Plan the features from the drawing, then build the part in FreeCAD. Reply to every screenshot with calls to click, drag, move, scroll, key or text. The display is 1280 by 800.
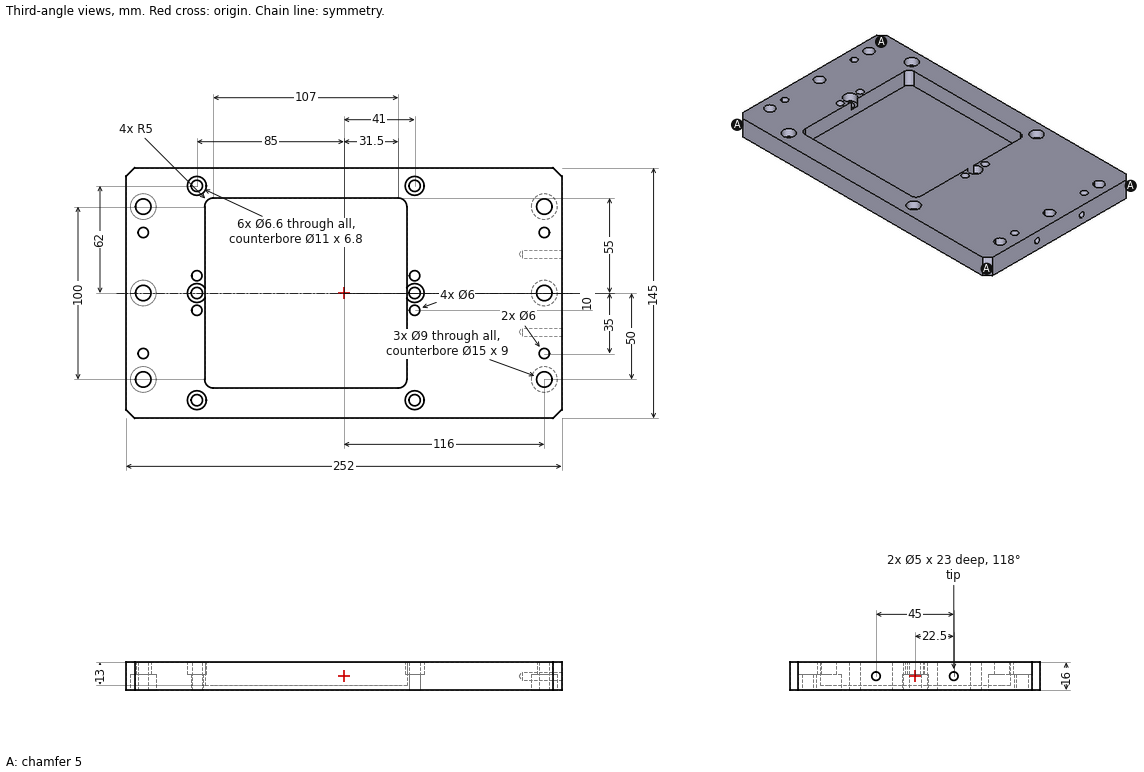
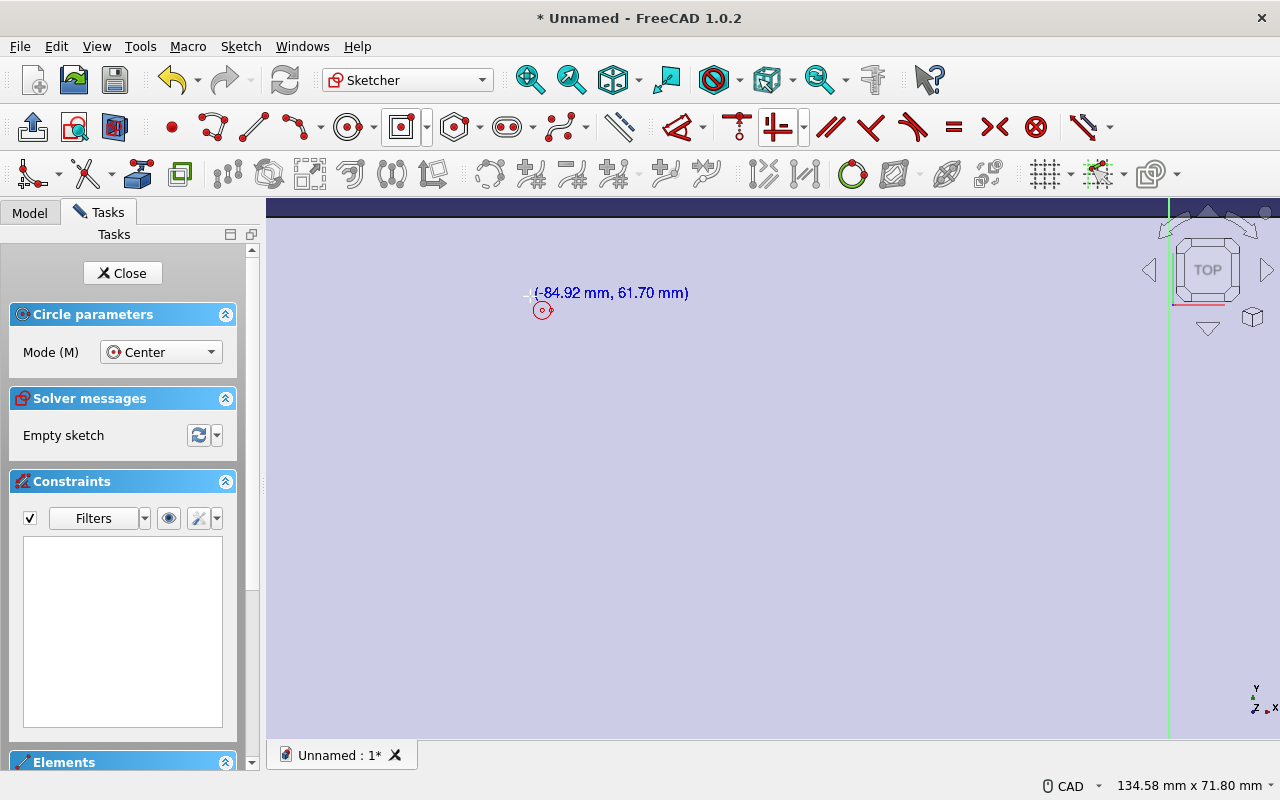
click(529, 296)
move(547, 279)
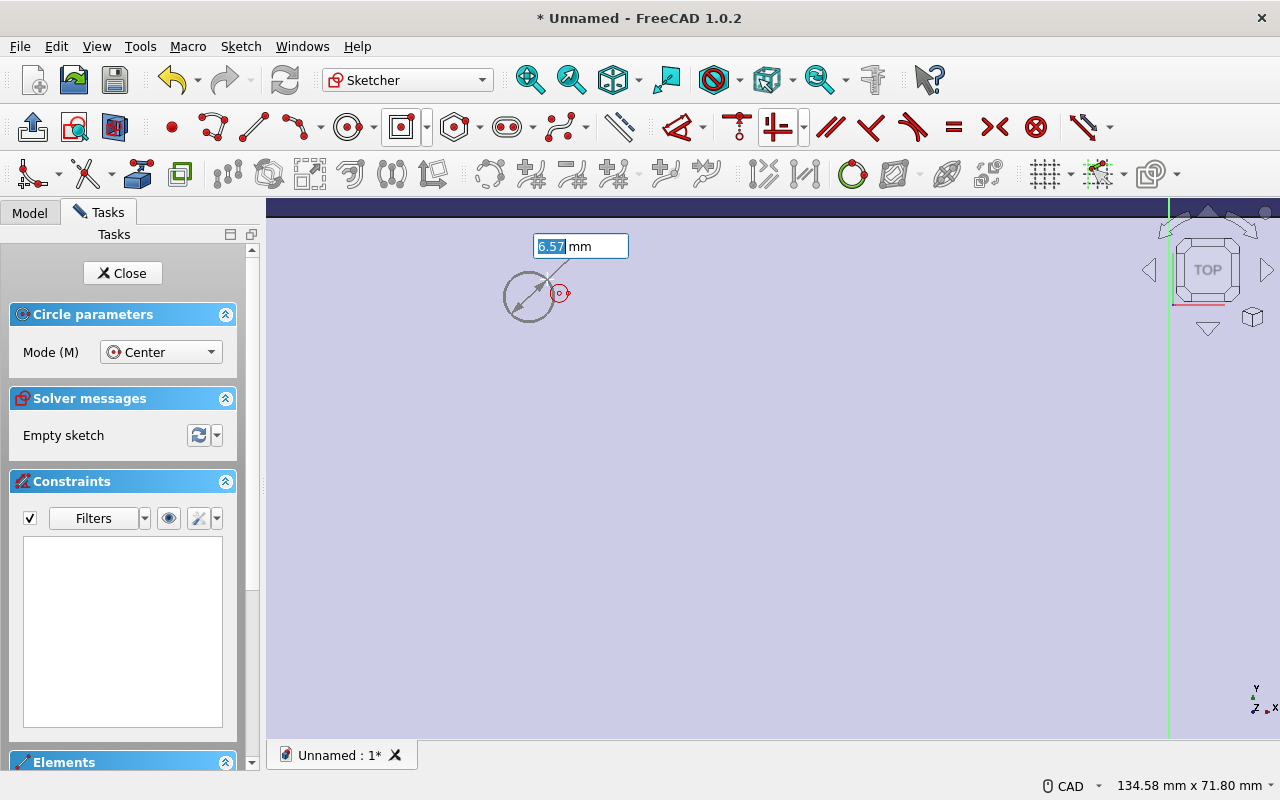
text(6.6)
key(Return)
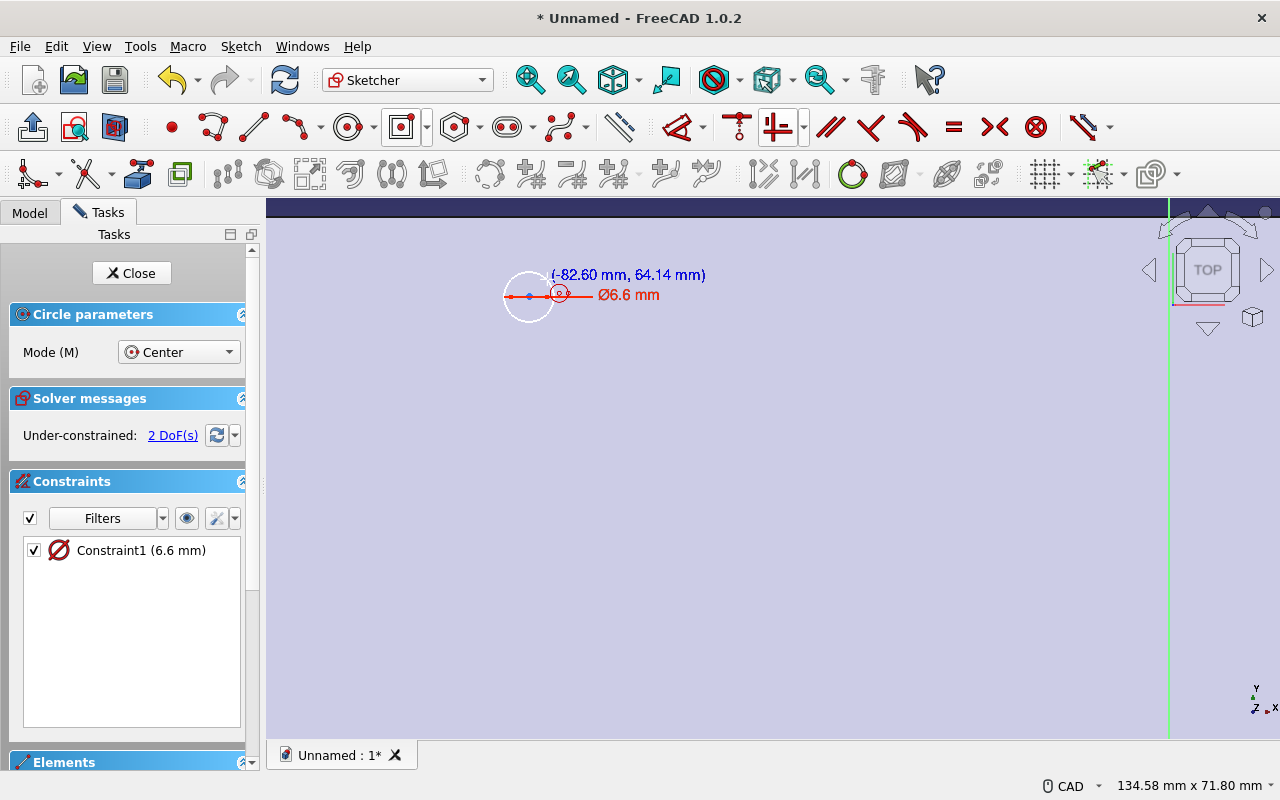
scroll(530, 297, down, 5)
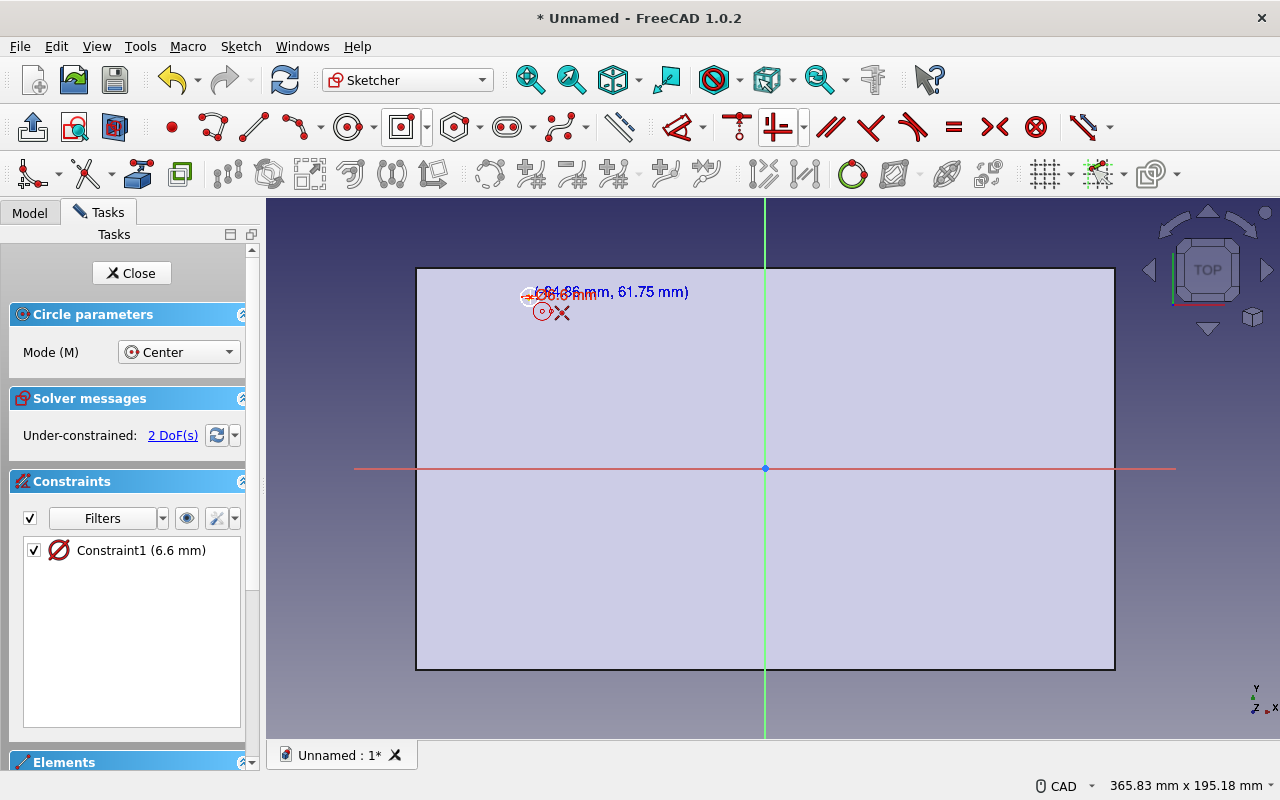
scroll(530, 469, up, 5)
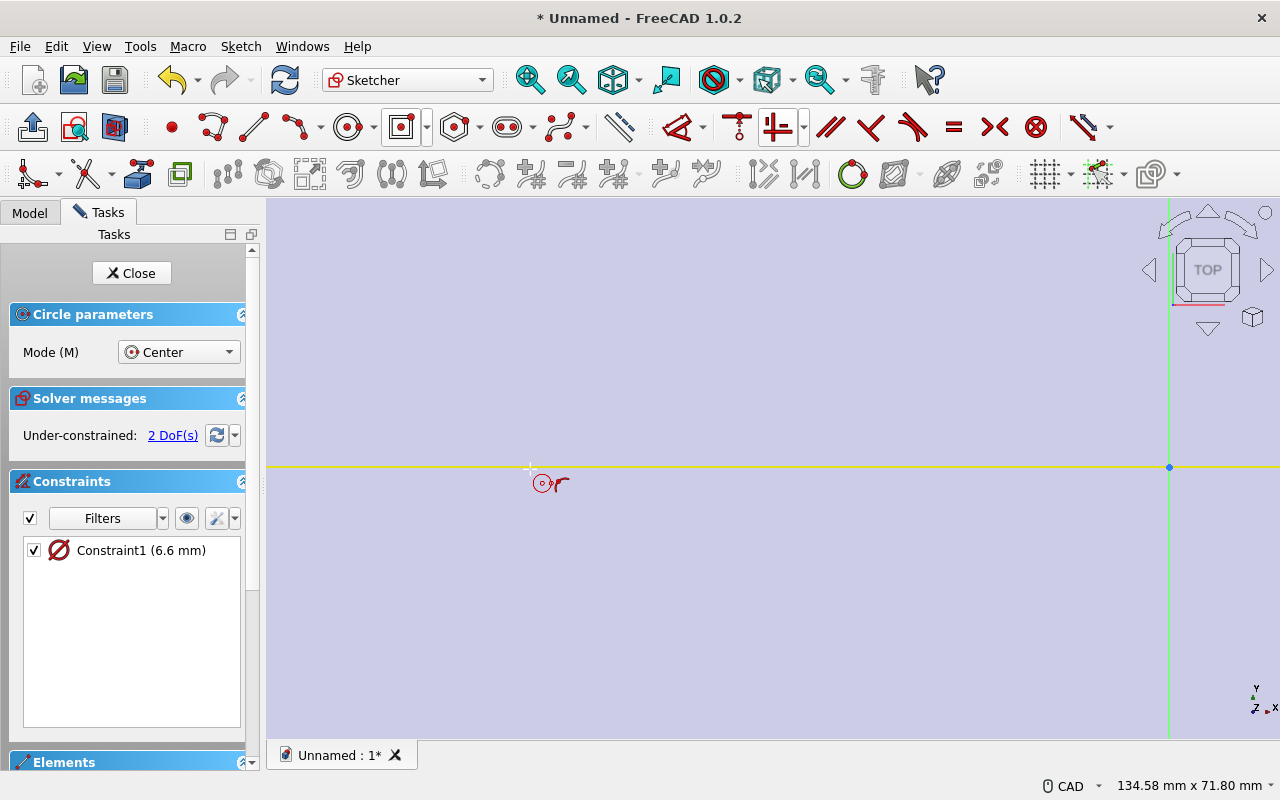
click(529, 467)
move(547, 450)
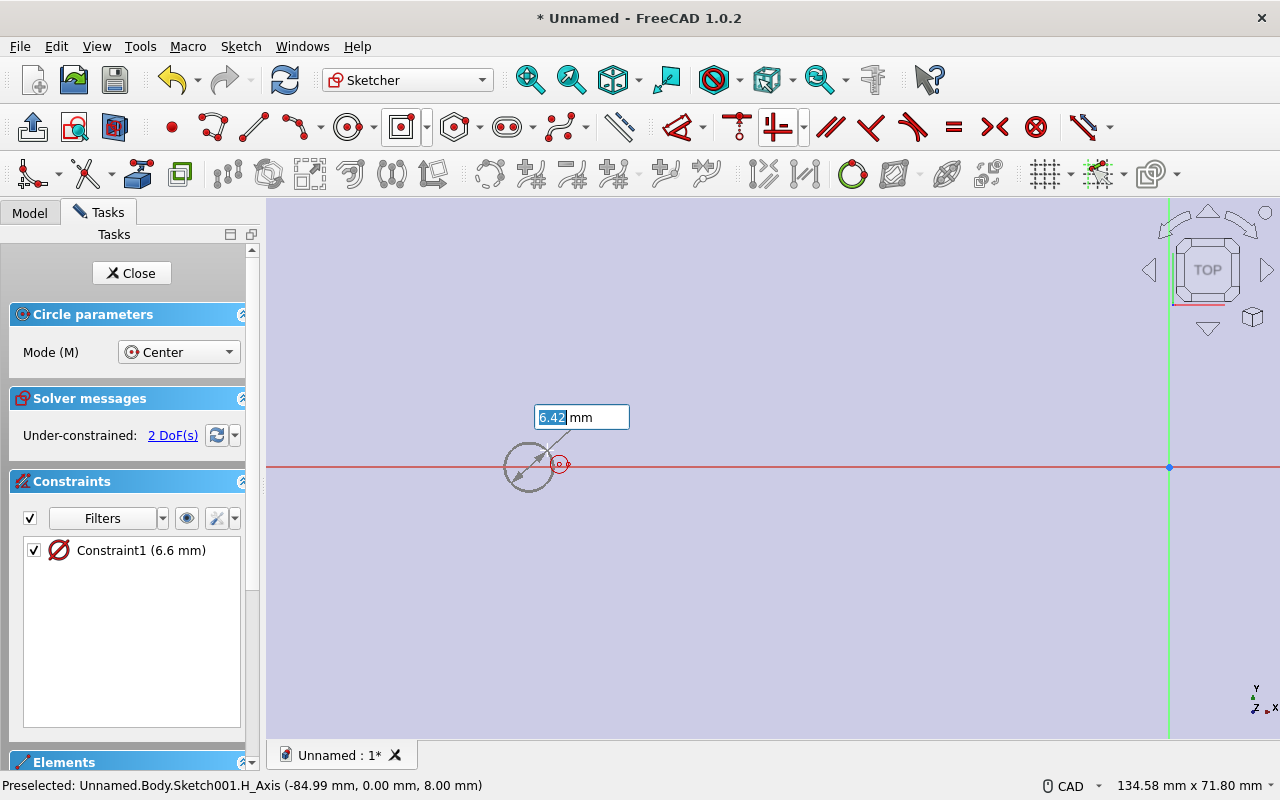
text(6.6)
key(Return)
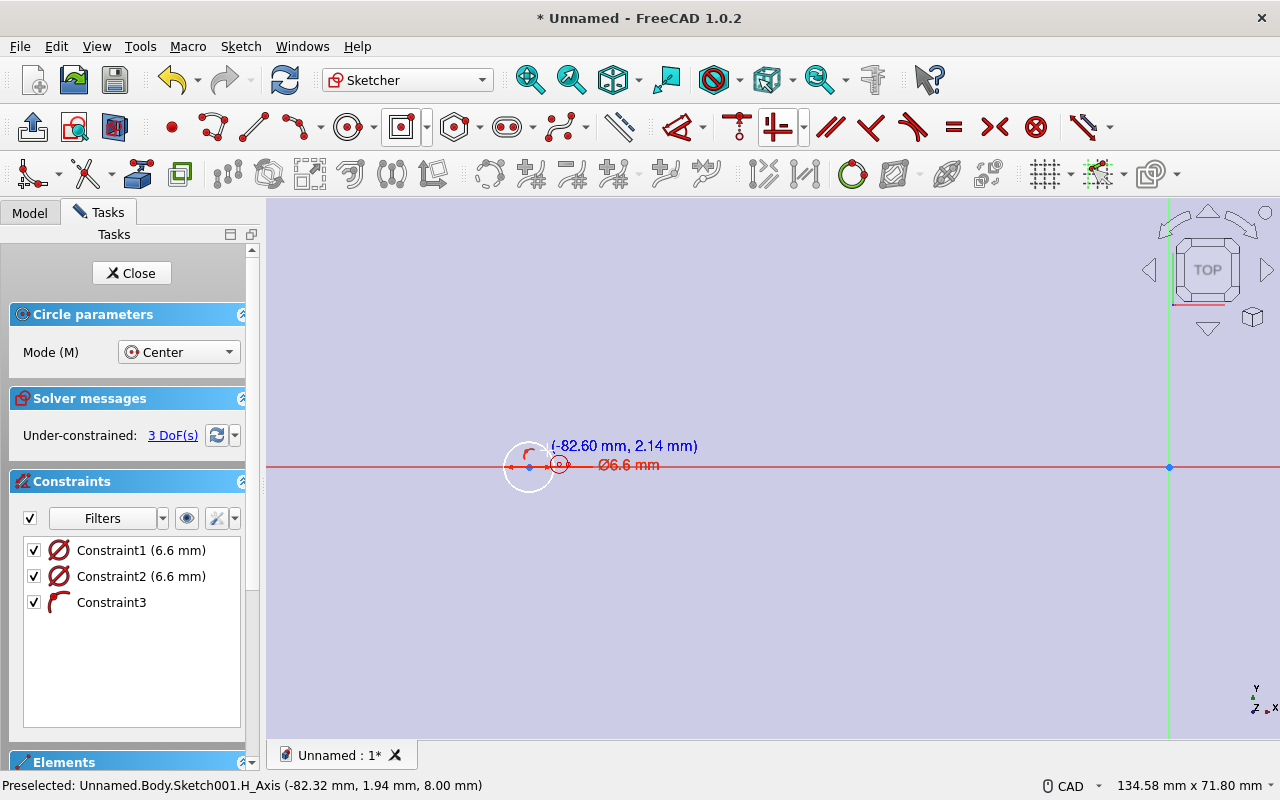
scroll(530, 469, down, 5)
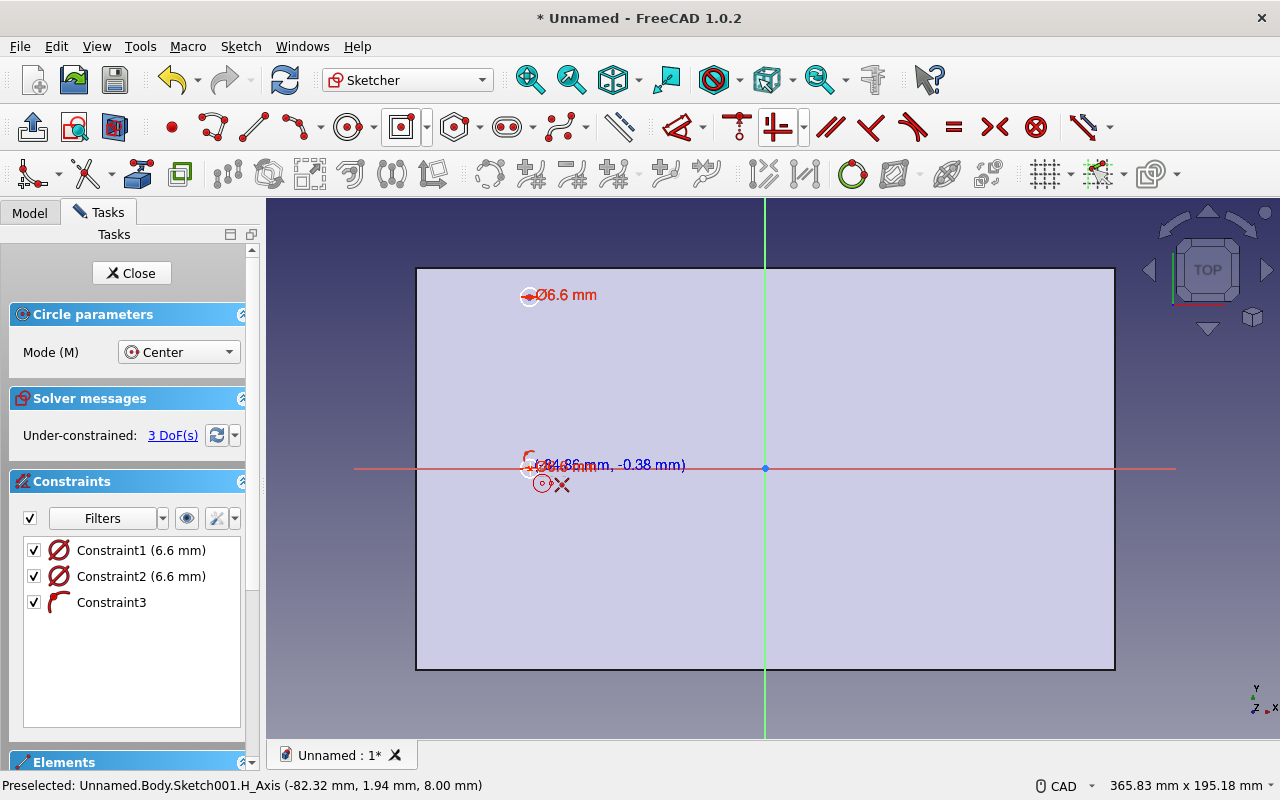
scroll(879, 297, up, 5)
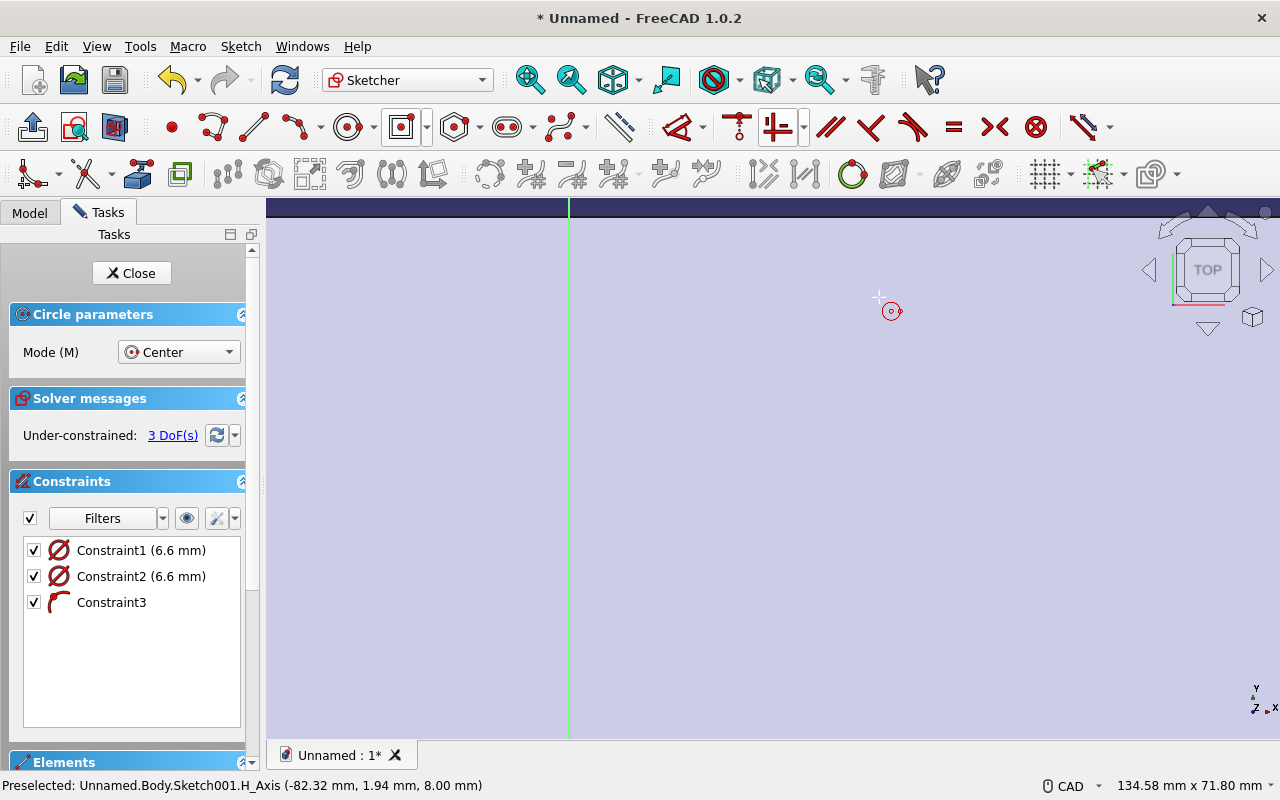
click(878, 296)
move(896, 279)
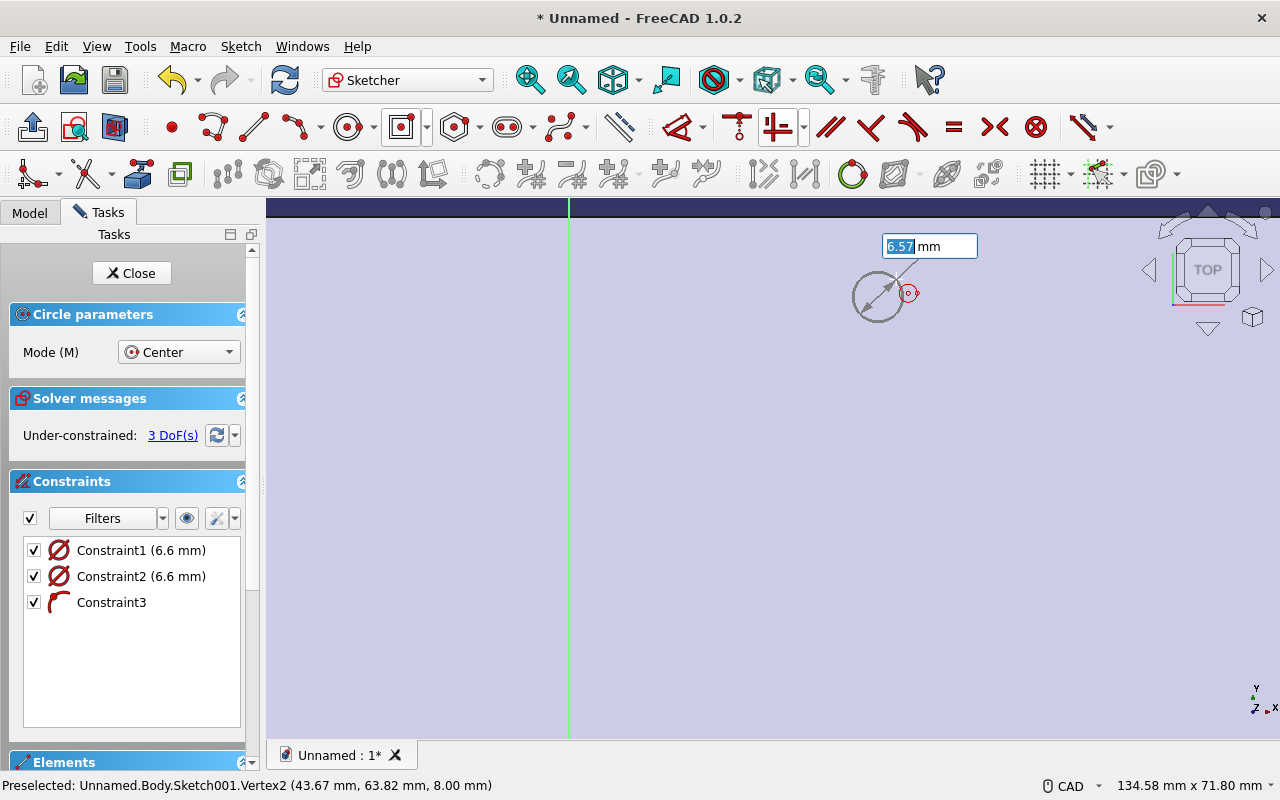
text(6.6)
key(Return)